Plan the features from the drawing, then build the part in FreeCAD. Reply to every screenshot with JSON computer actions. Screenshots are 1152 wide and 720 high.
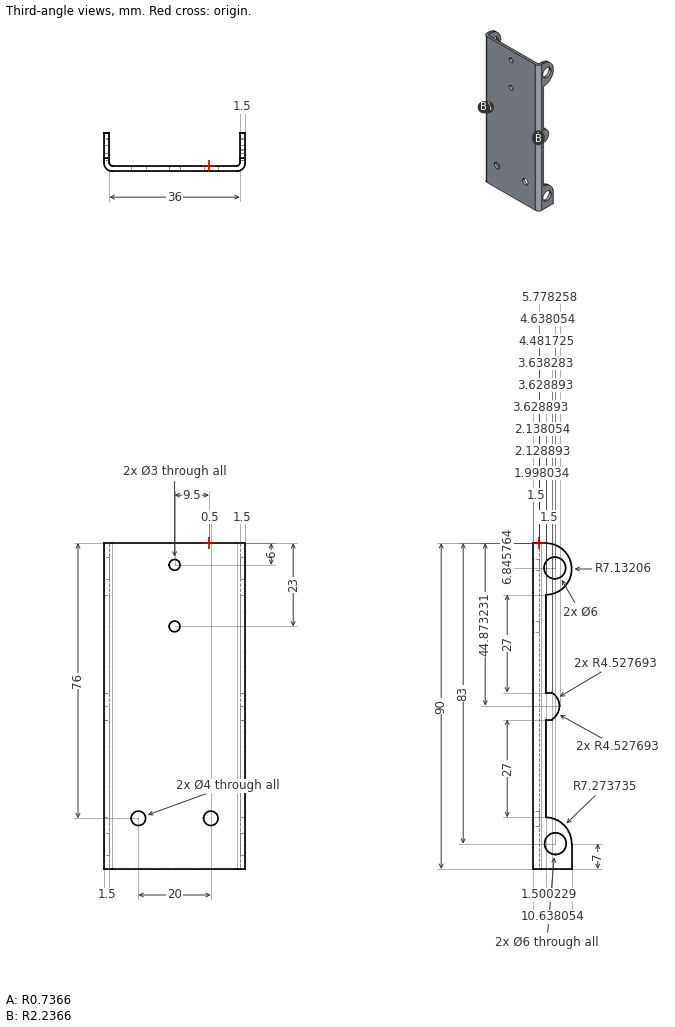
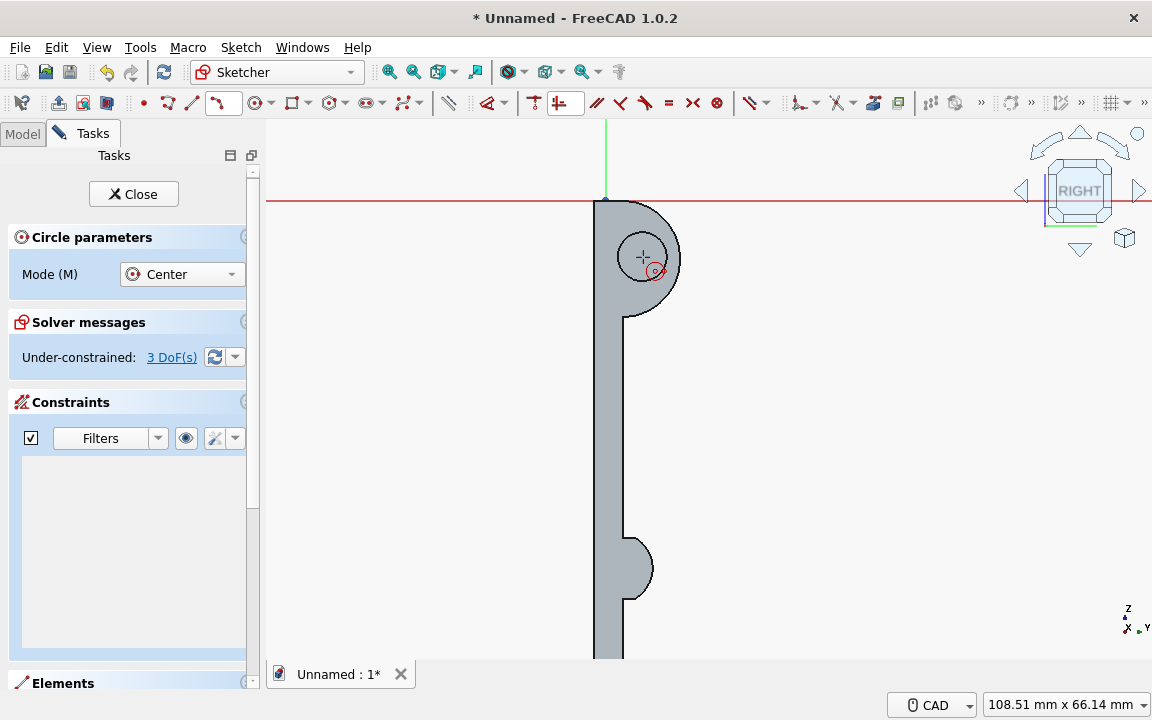
{"action": "left_click", "coordinate": [642, 257]}
{"action": "left_click", "coordinate": [660, 239]}
{"action": "key", "text": "Escape"}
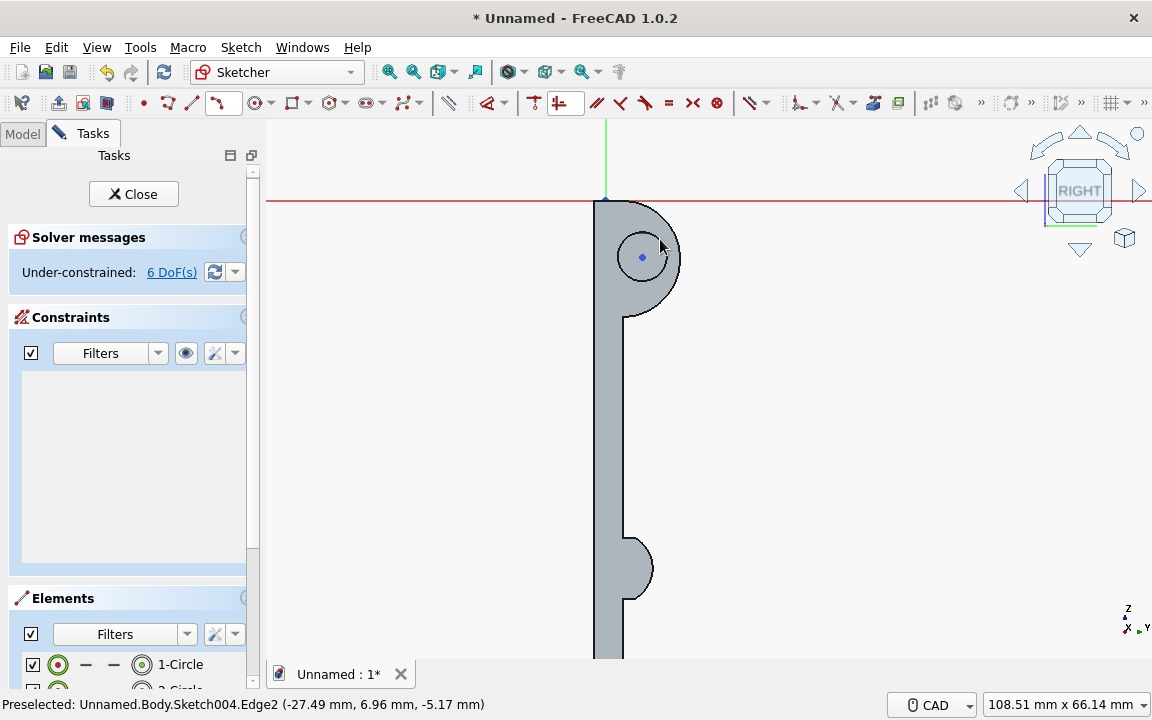
{"action": "scroll", "coordinate": [643, 256], "scroll_direction": "down", "scroll_amount": 4}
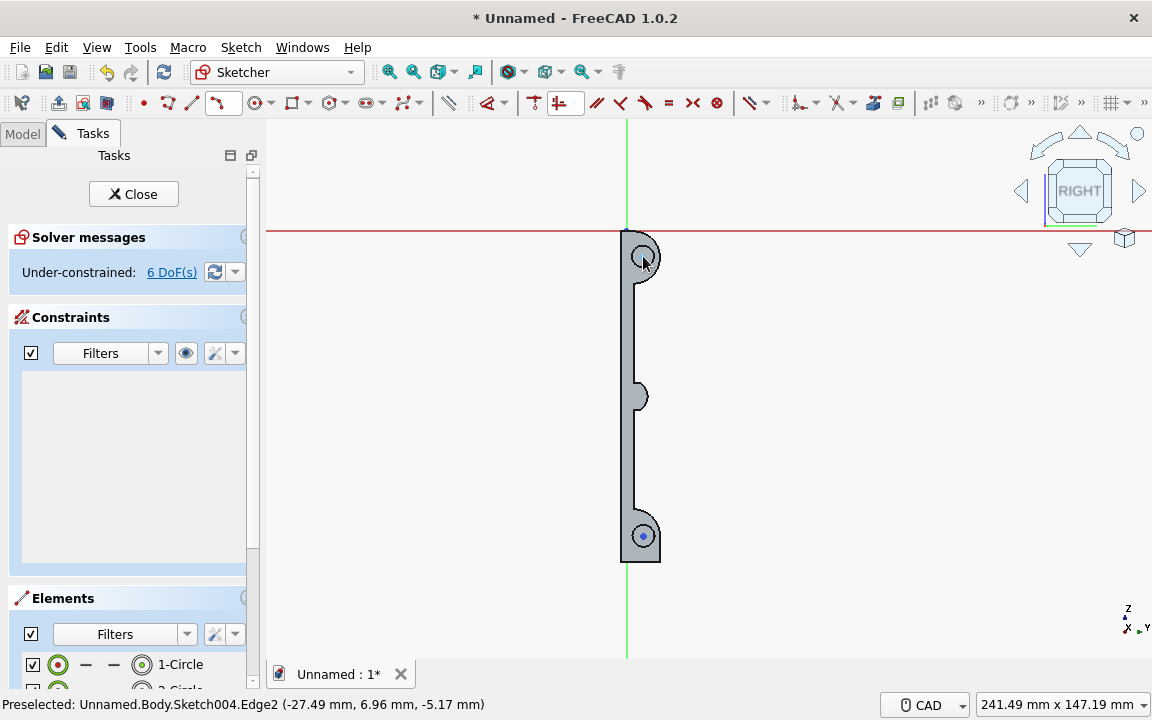
{"action": "left_click", "coordinate": [651, 528]}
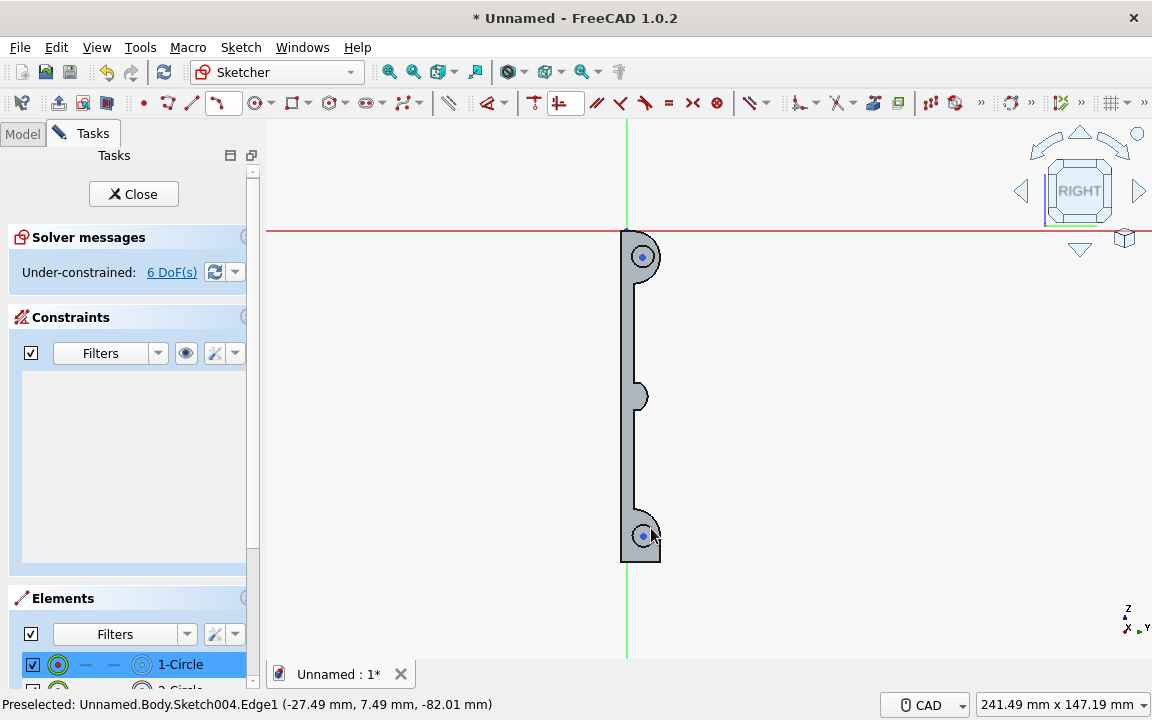
{"action": "left_click", "coordinate": [651, 249]}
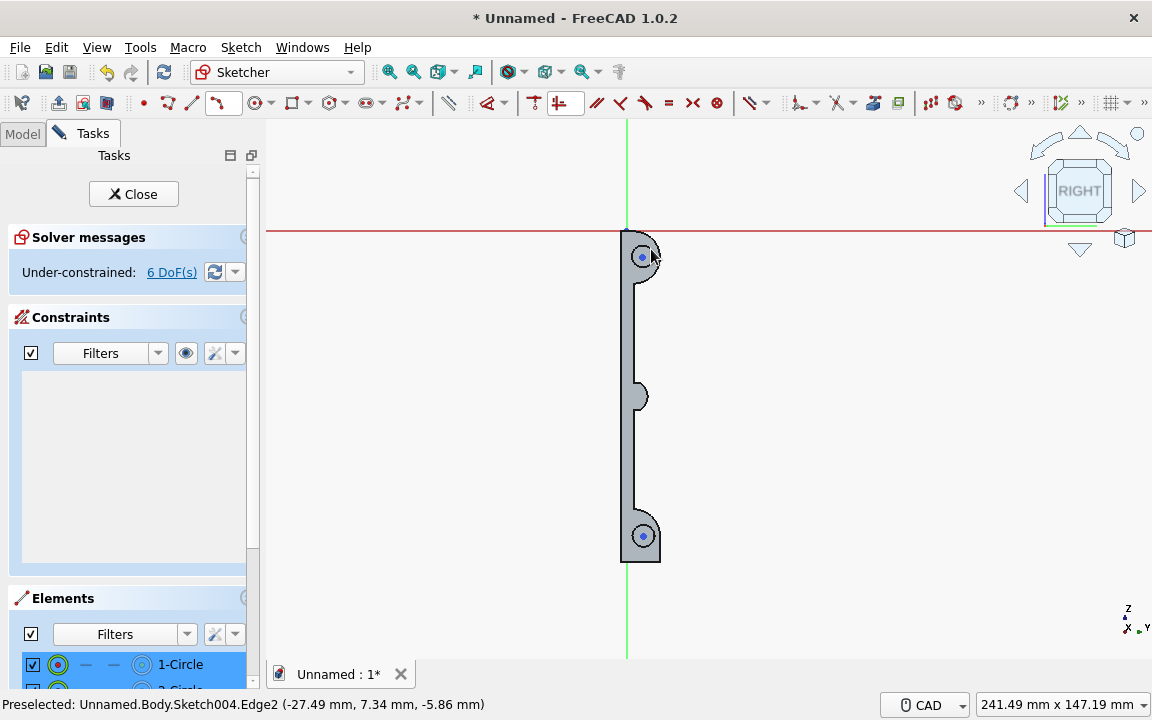
{"action": "key", "text": "e"}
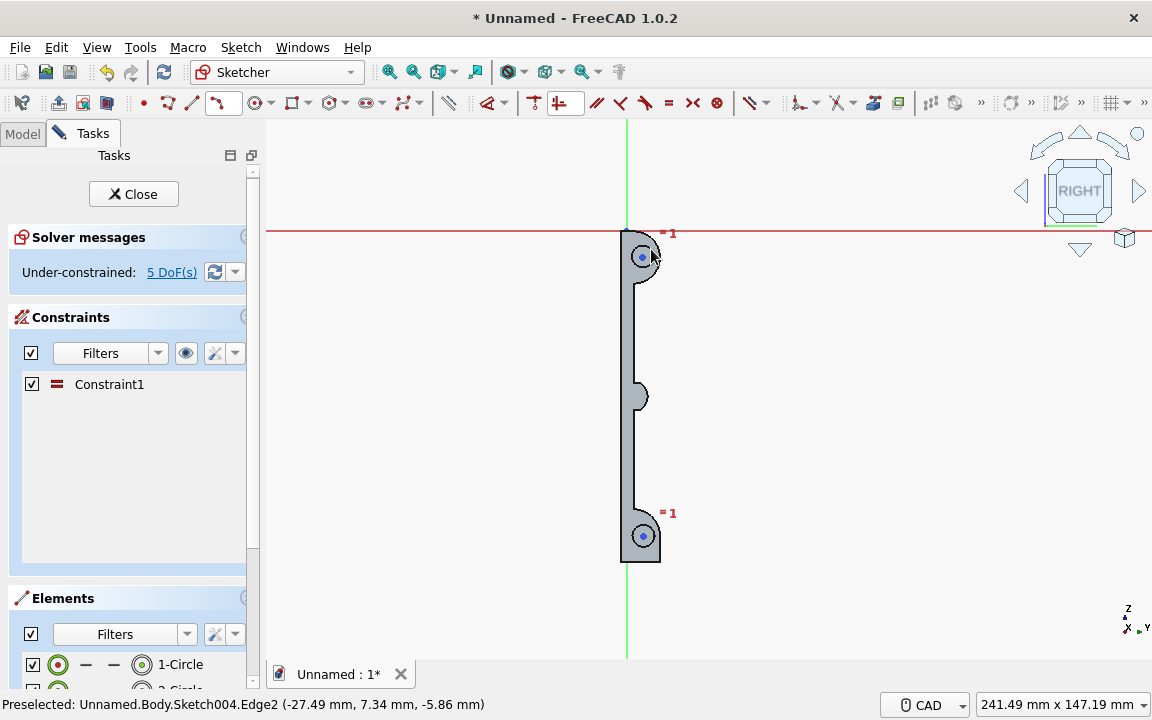
{"action": "key", "text": "d"}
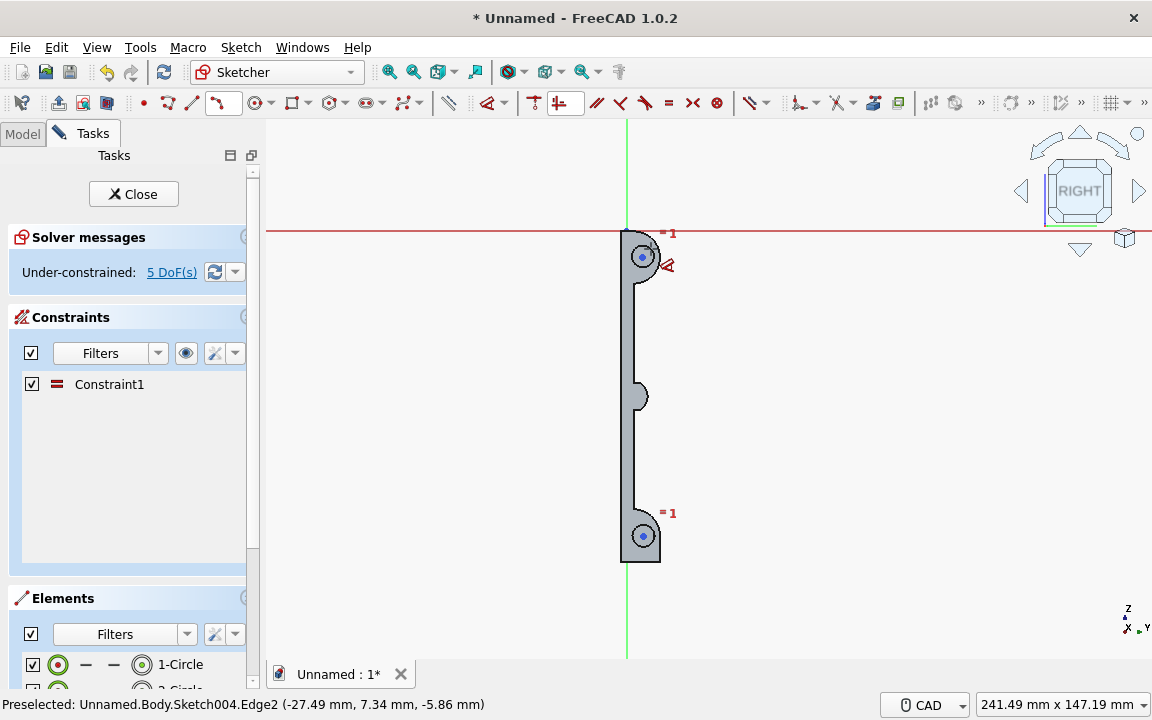
{"action": "scroll", "coordinate": [651, 528], "scroll_direction": "up", "scroll_amount": 3}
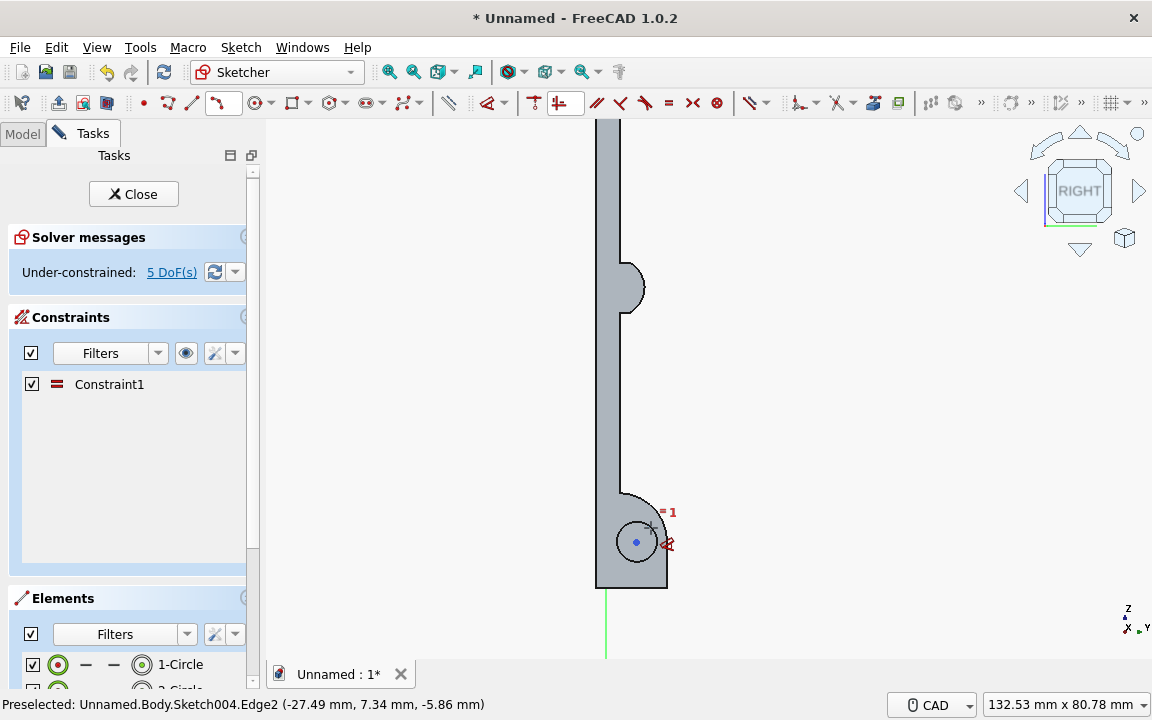
{"action": "left_click", "coordinate": [651, 528]}
{"action": "left_click", "coordinate": [673, 505]}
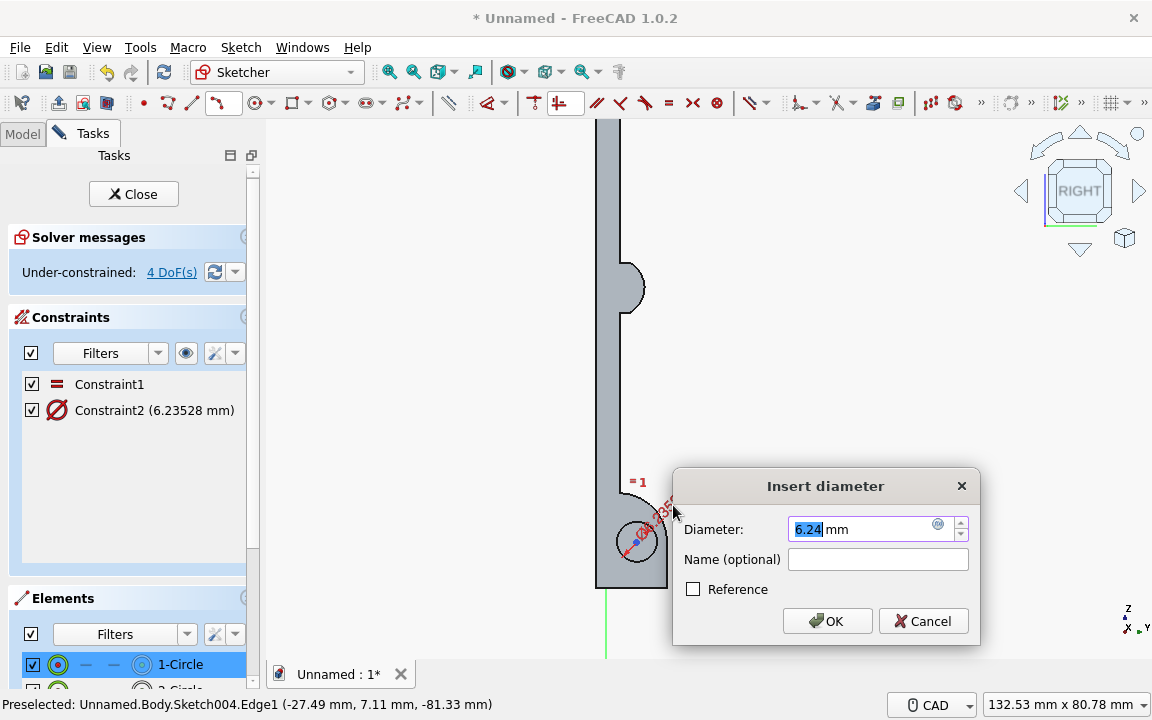
{"action": "type", "text": "6"}
{"action": "key", "text": "Return"}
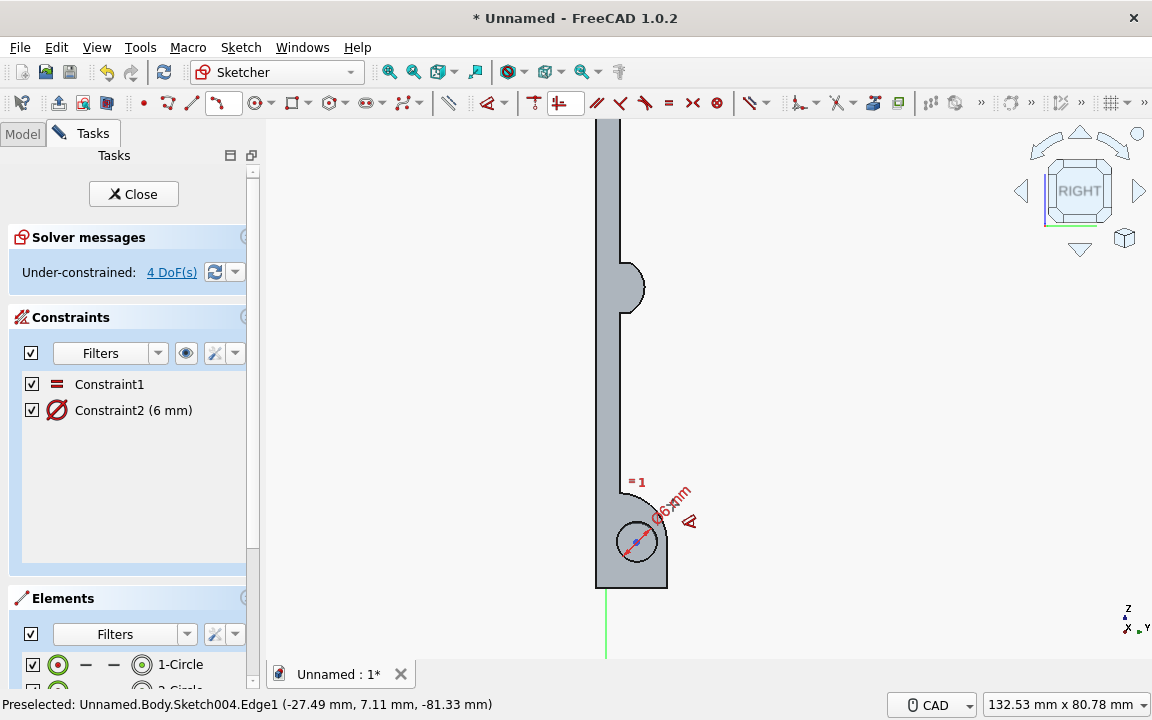
{"action": "left_click", "coordinate": [637, 543]}
{"action": "left_click", "coordinate": [572, 345]}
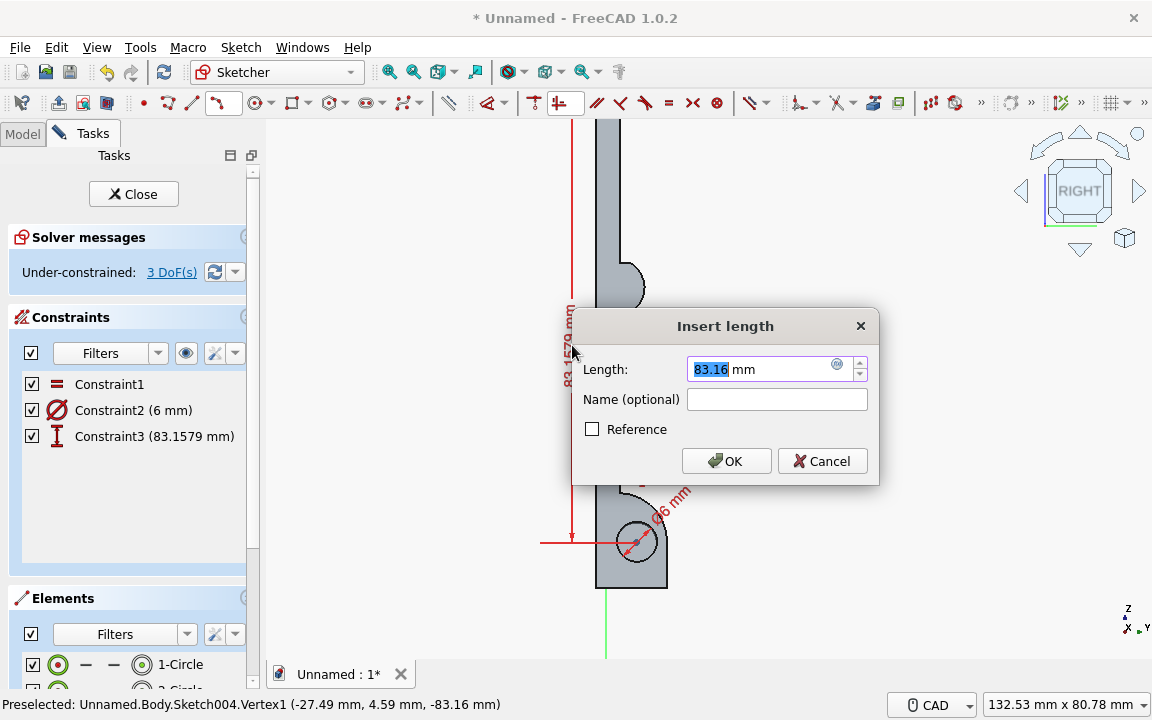
{"action": "type", "text": "83"}
{"action": "key", "text": "Return"}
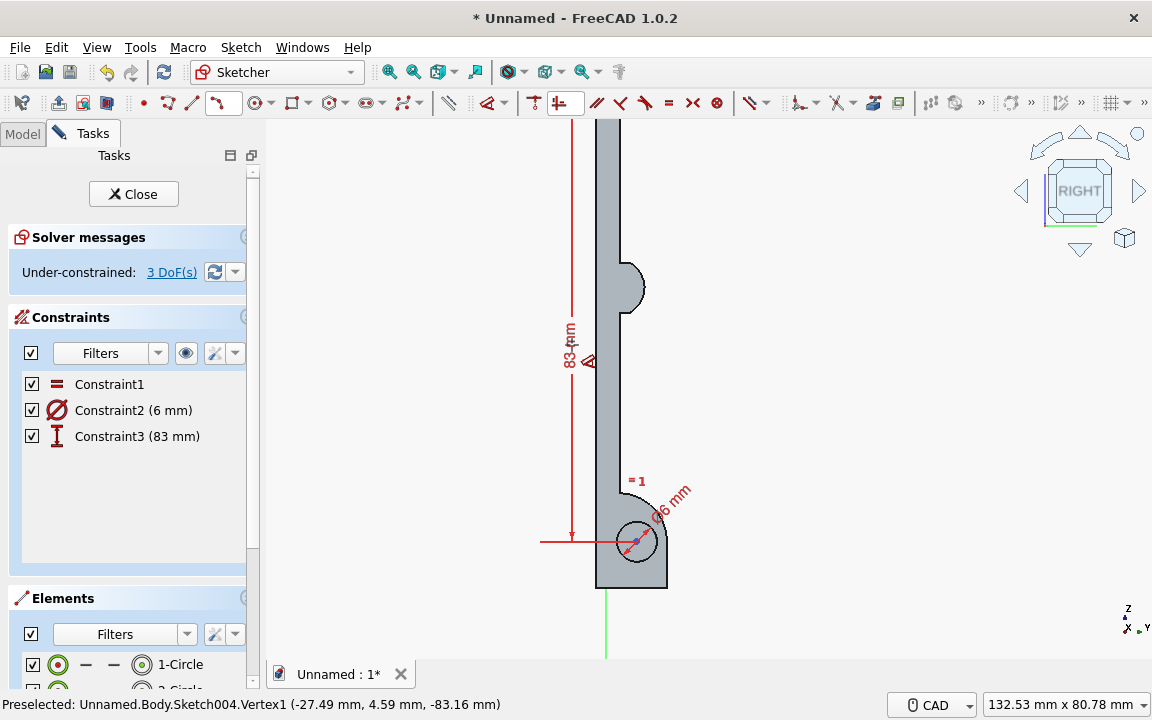
{"action": "scroll", "coordinate": [637, 542], "scroll_direction": "up", "scroll_amount": 2}